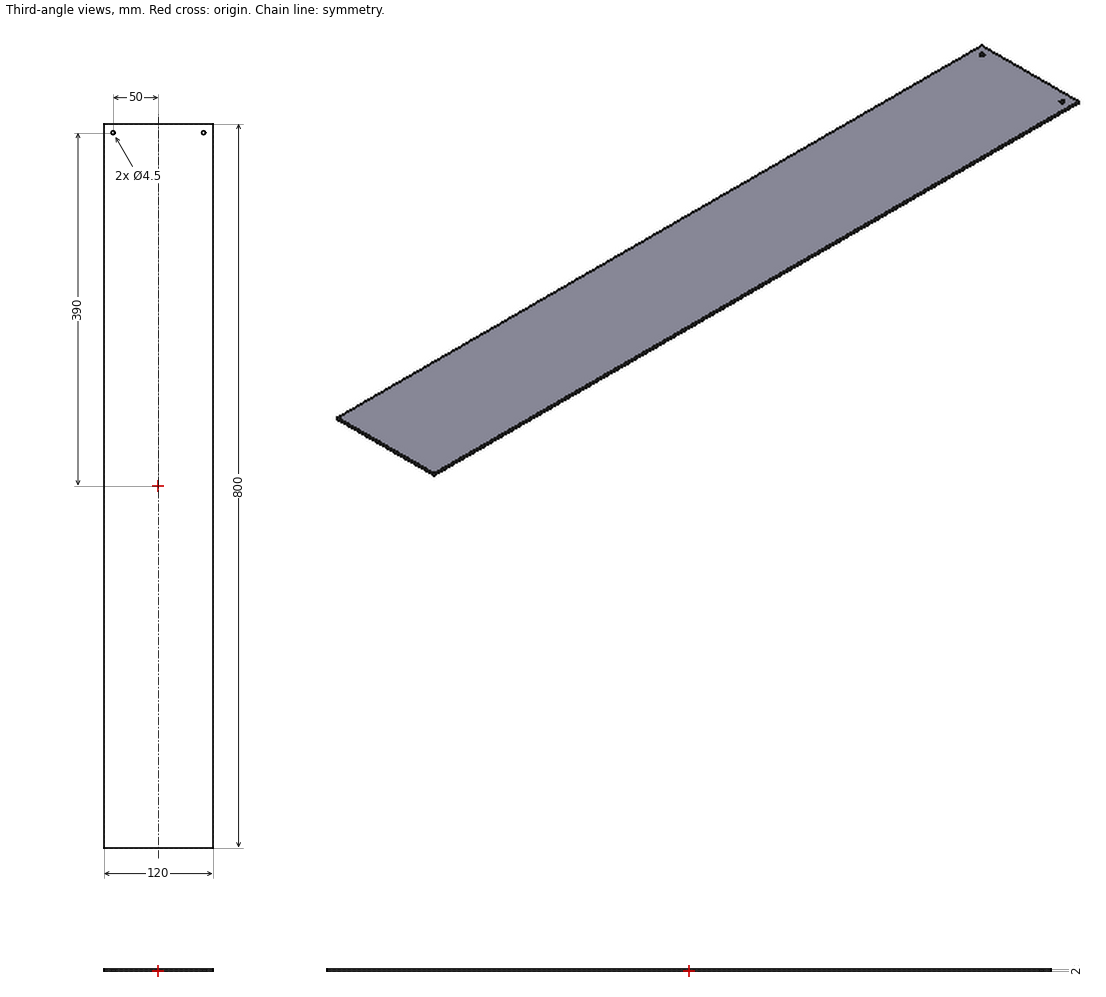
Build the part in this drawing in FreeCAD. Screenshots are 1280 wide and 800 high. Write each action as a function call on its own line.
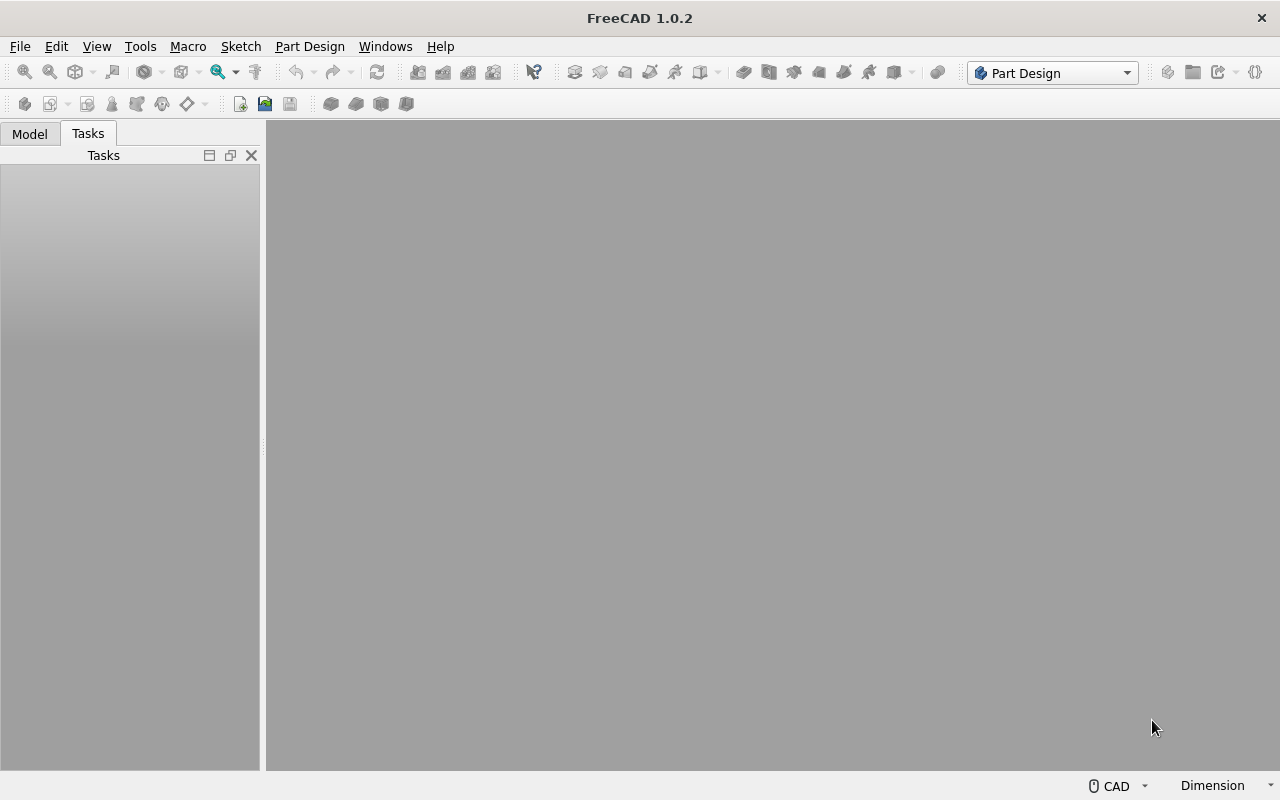
key(ctrl+n)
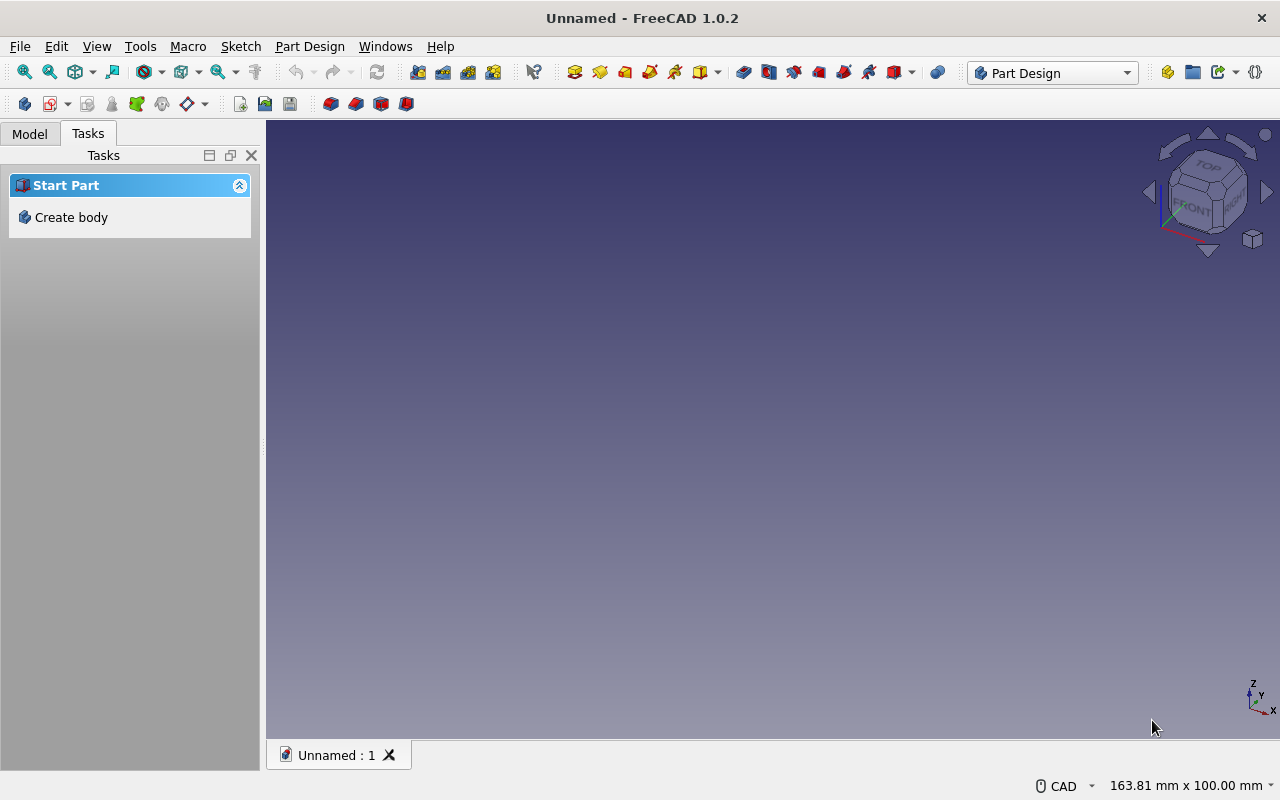
click(50, 104)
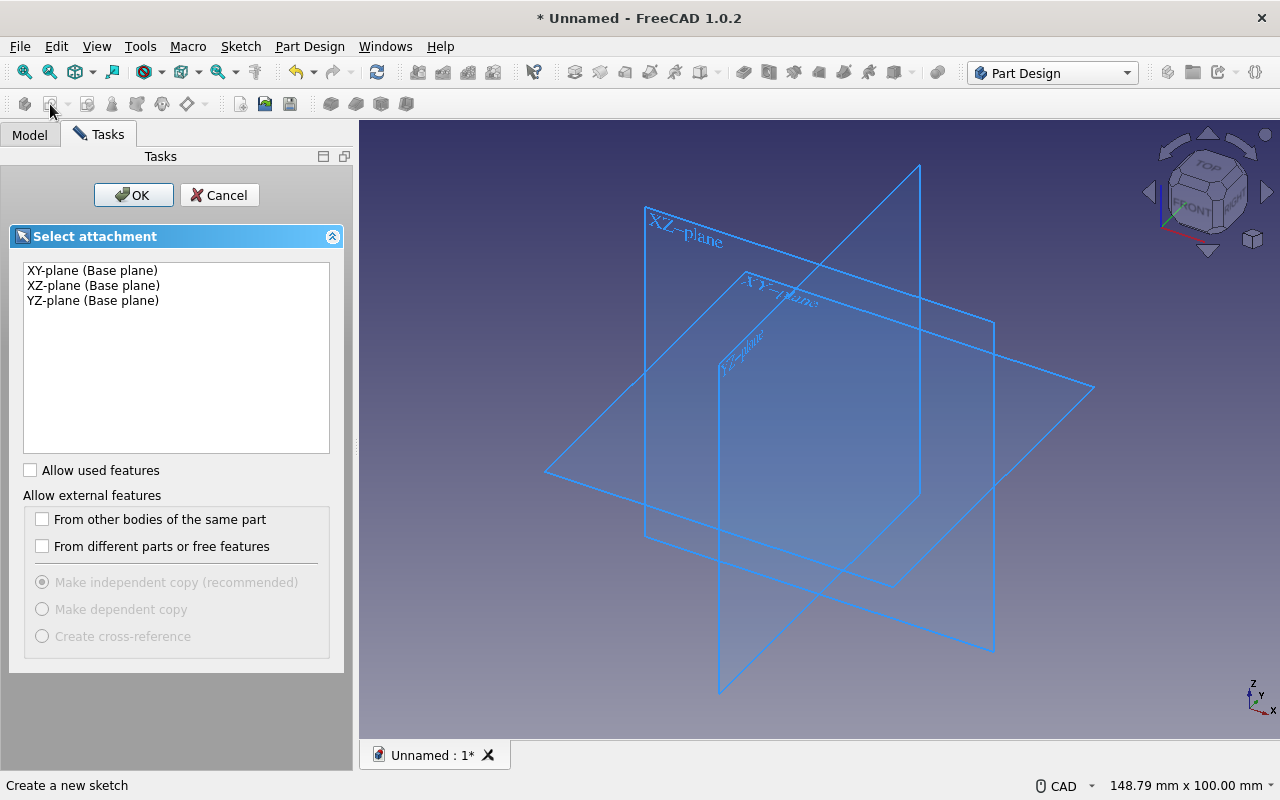
click(84, 270)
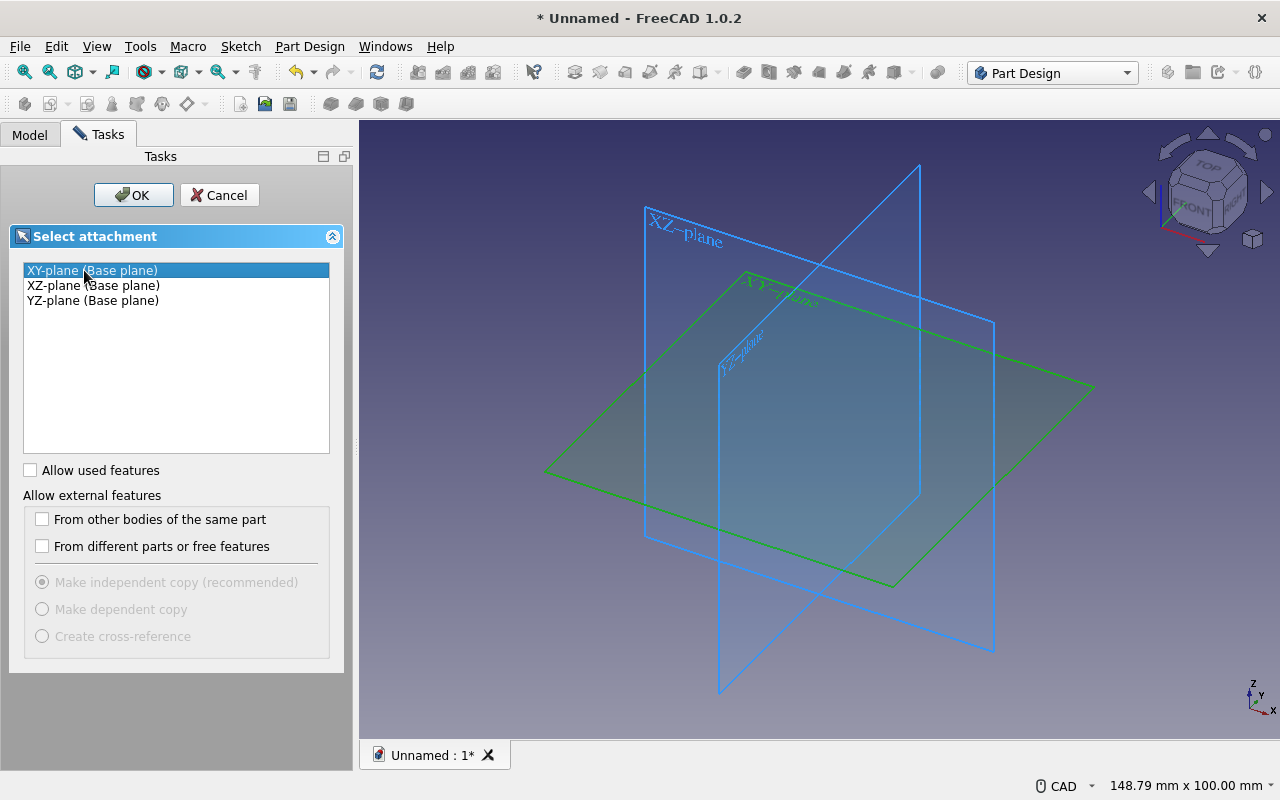
click(134, 195)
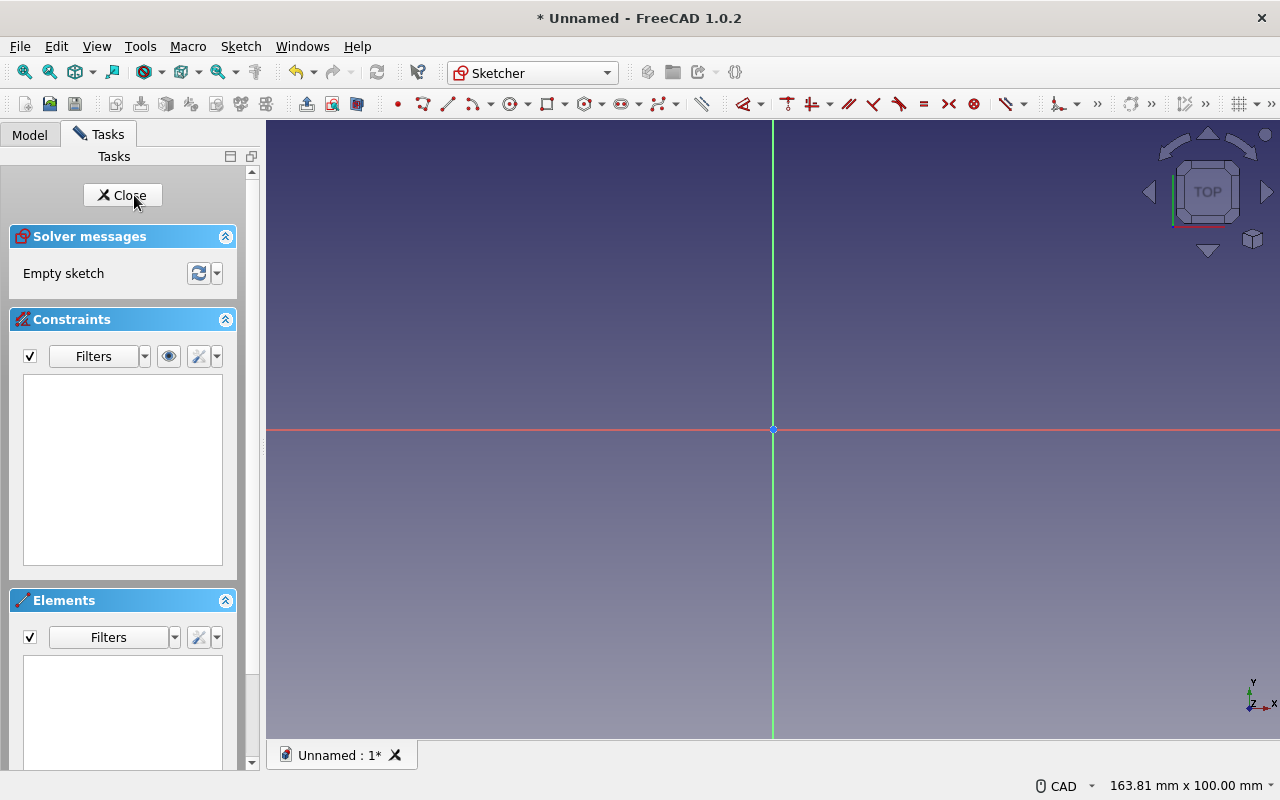
scroll(699, 430, down, 13)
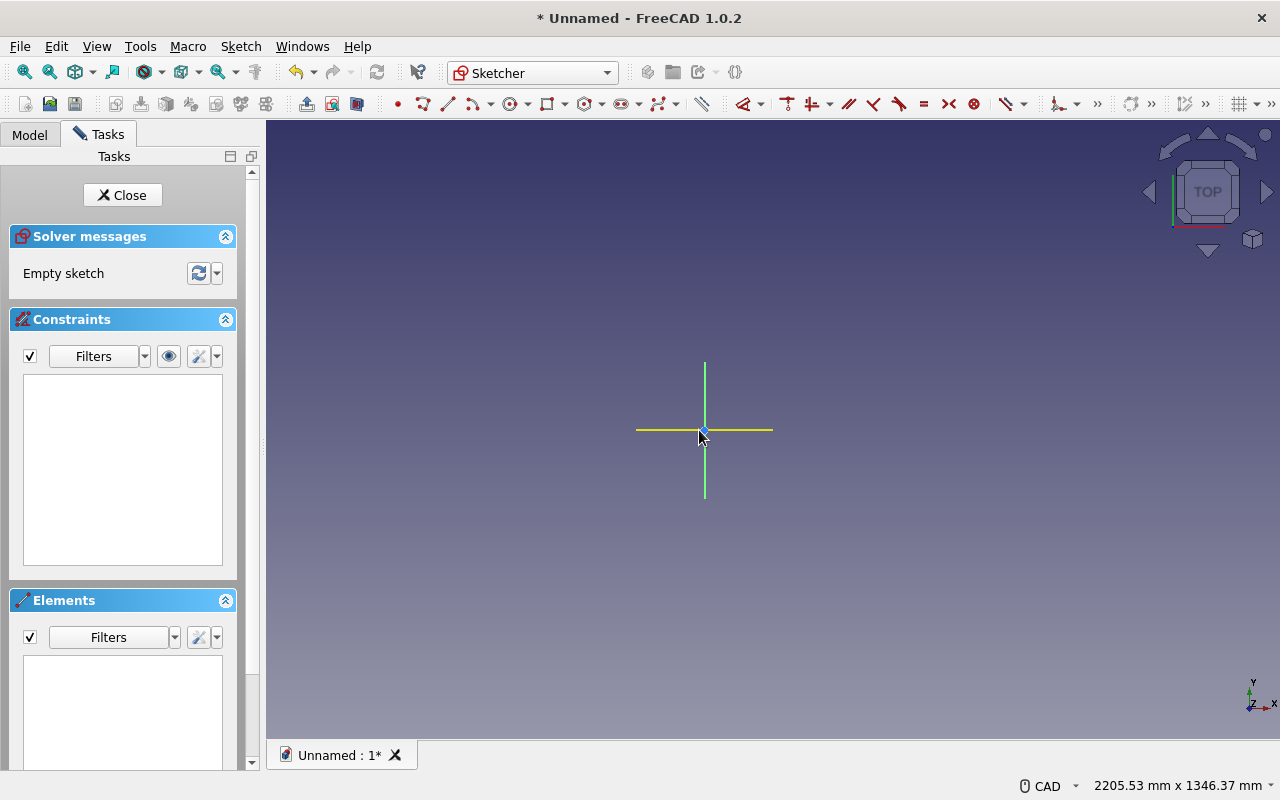
click(564, 104)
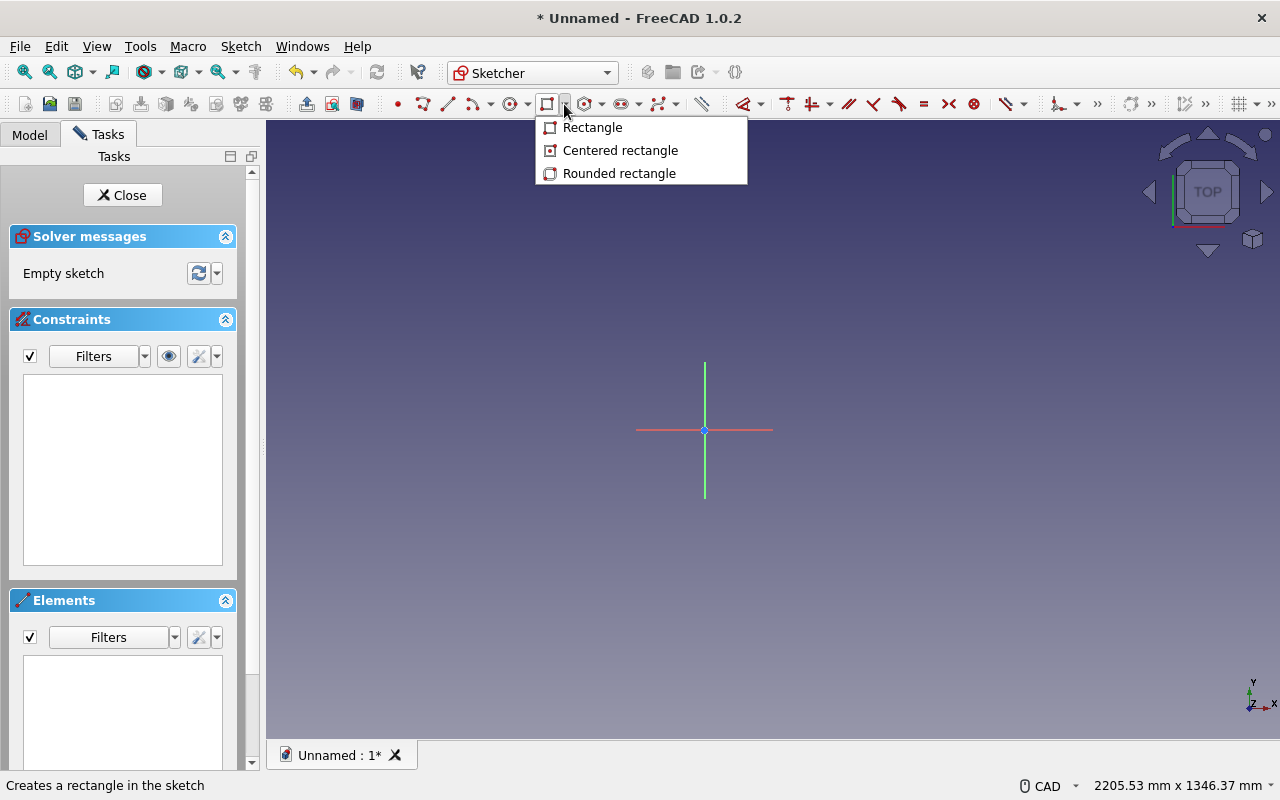
click(642, 150)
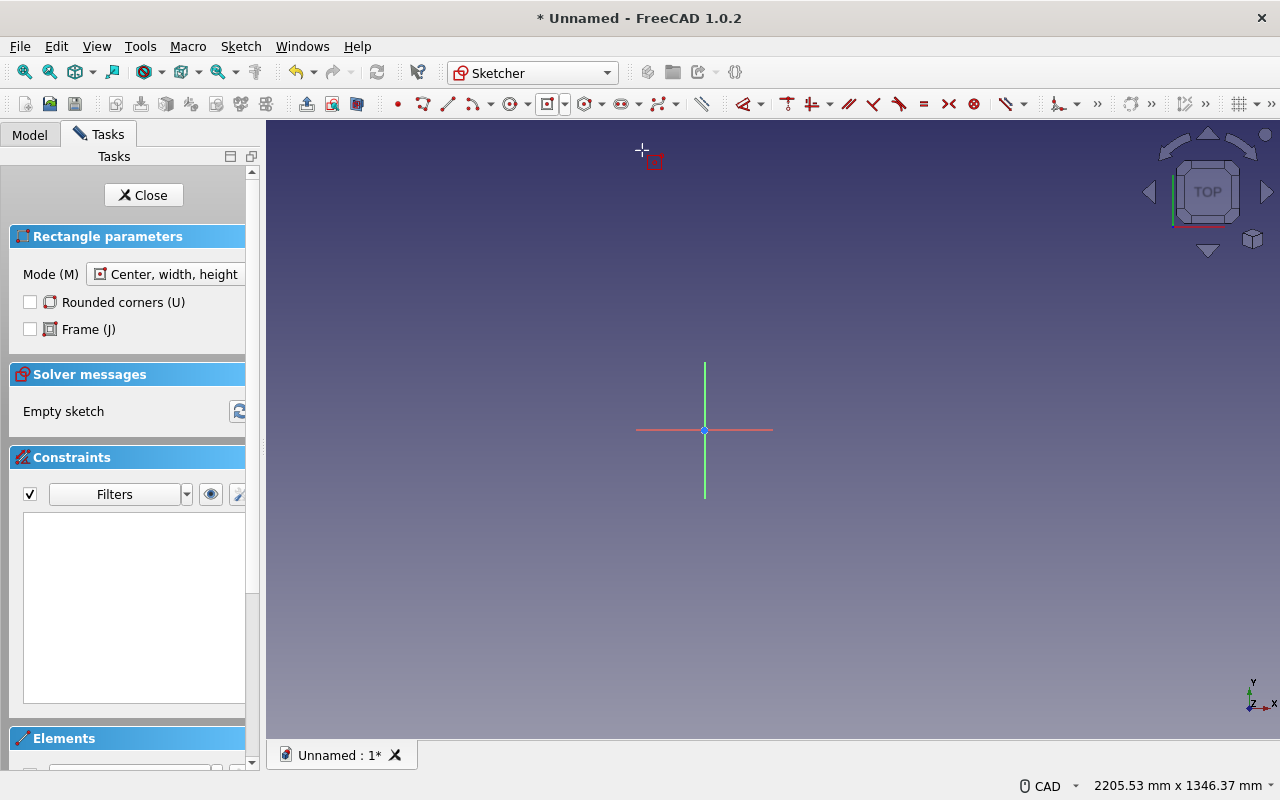
click(705, 430)
move(732, 247)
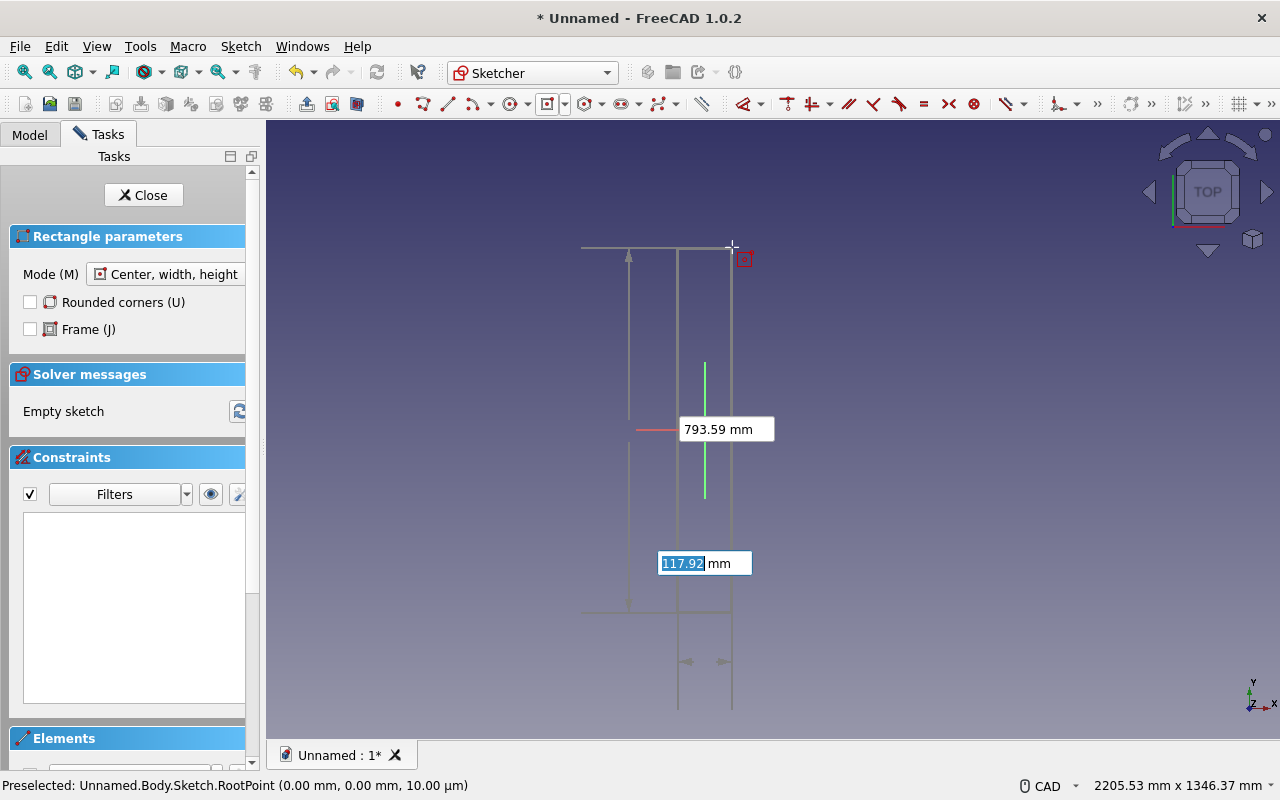
text(120)
key(Tab)
text(800)
key(Return)
key(Escape)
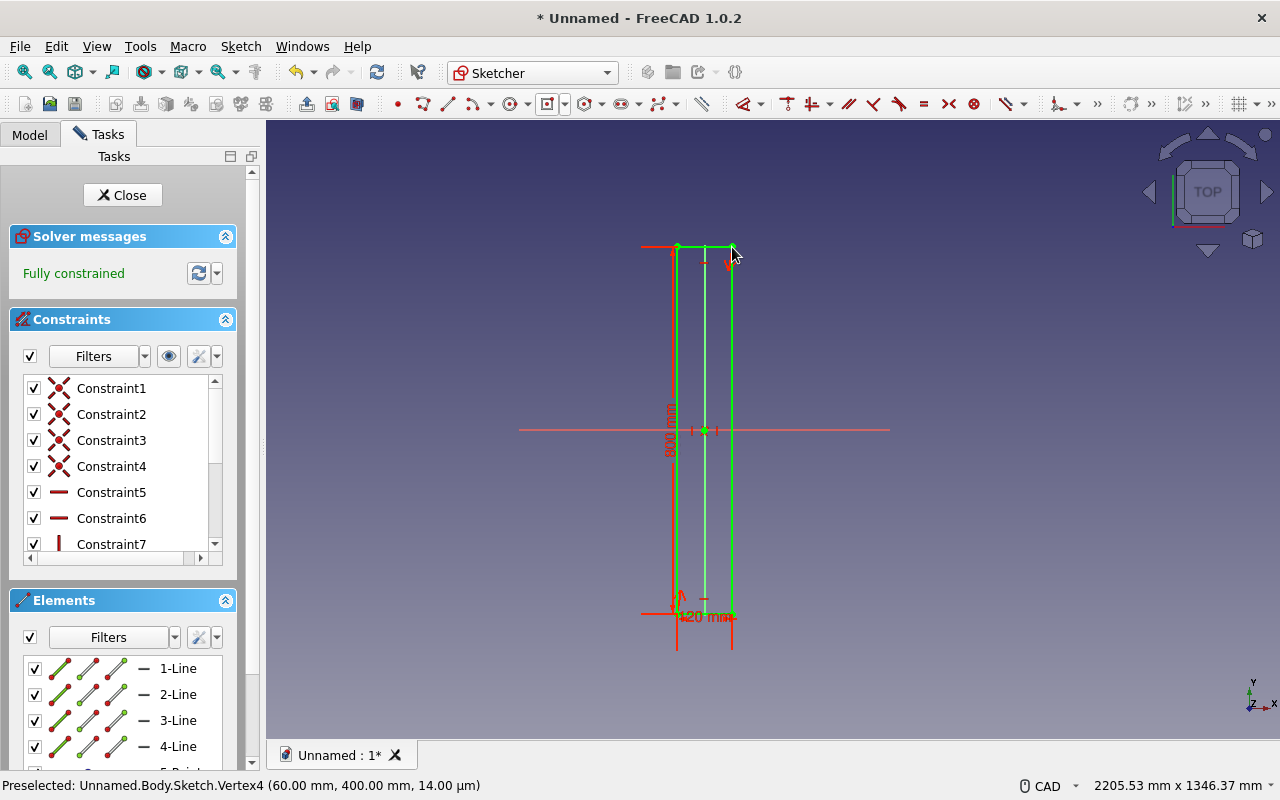
click(123, 195)